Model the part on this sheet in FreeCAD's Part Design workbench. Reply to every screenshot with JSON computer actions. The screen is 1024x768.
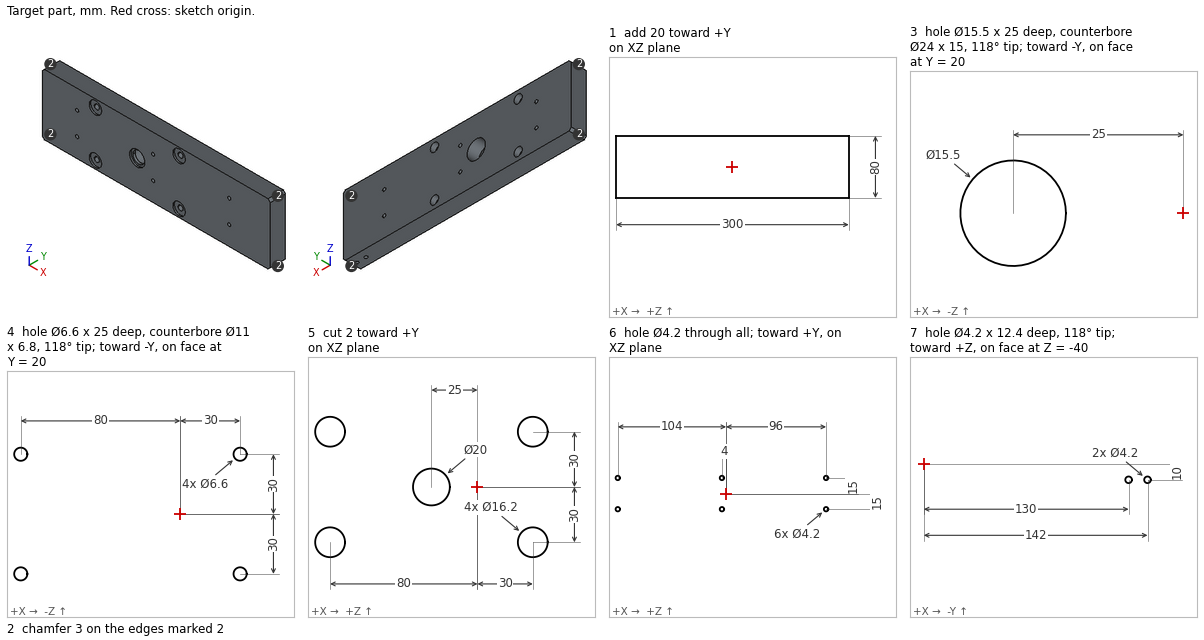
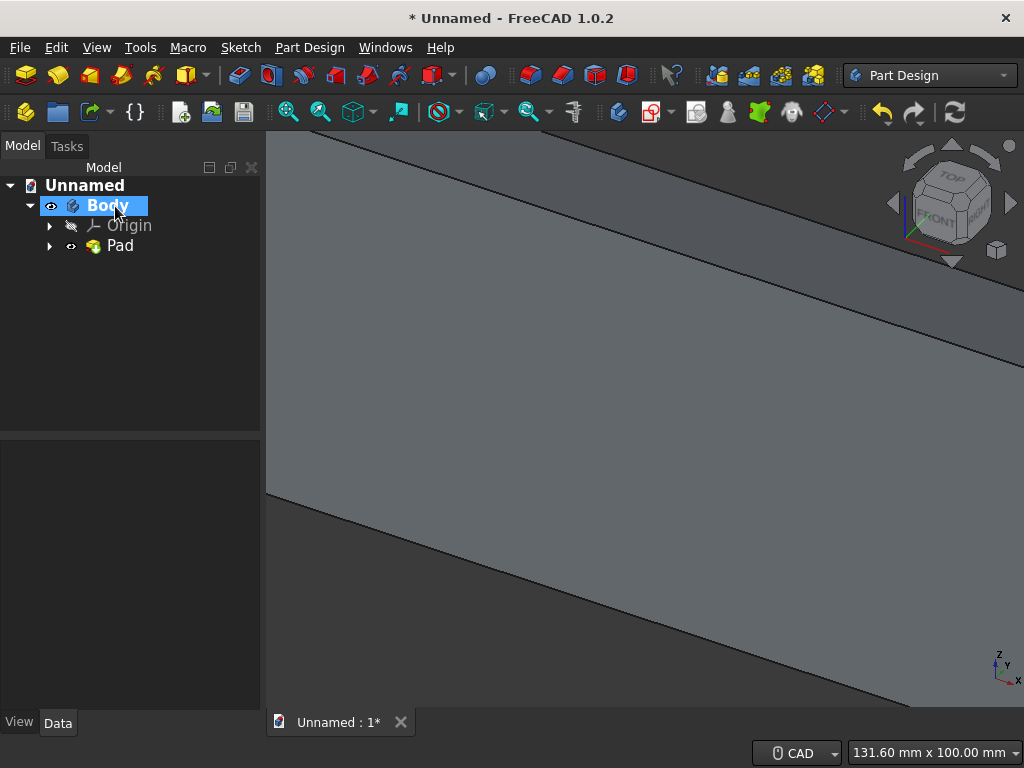
{"action": "left_click", "coordinate": [290, 112]}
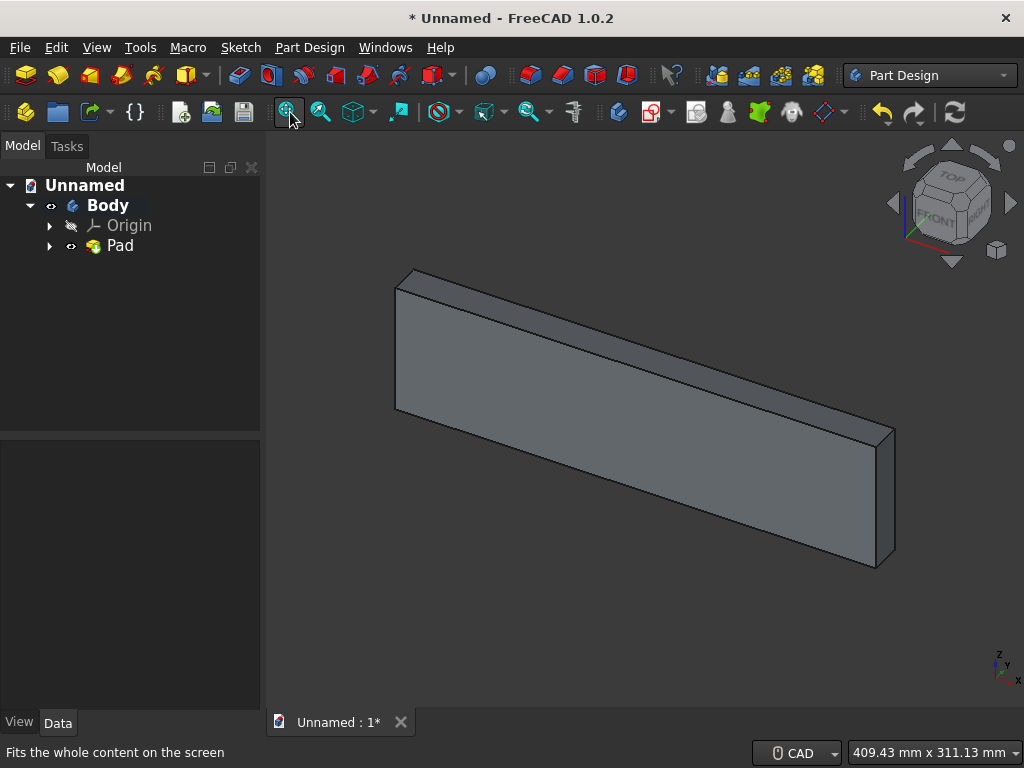
{"action": "left_click", "coordinate": [885, 437]}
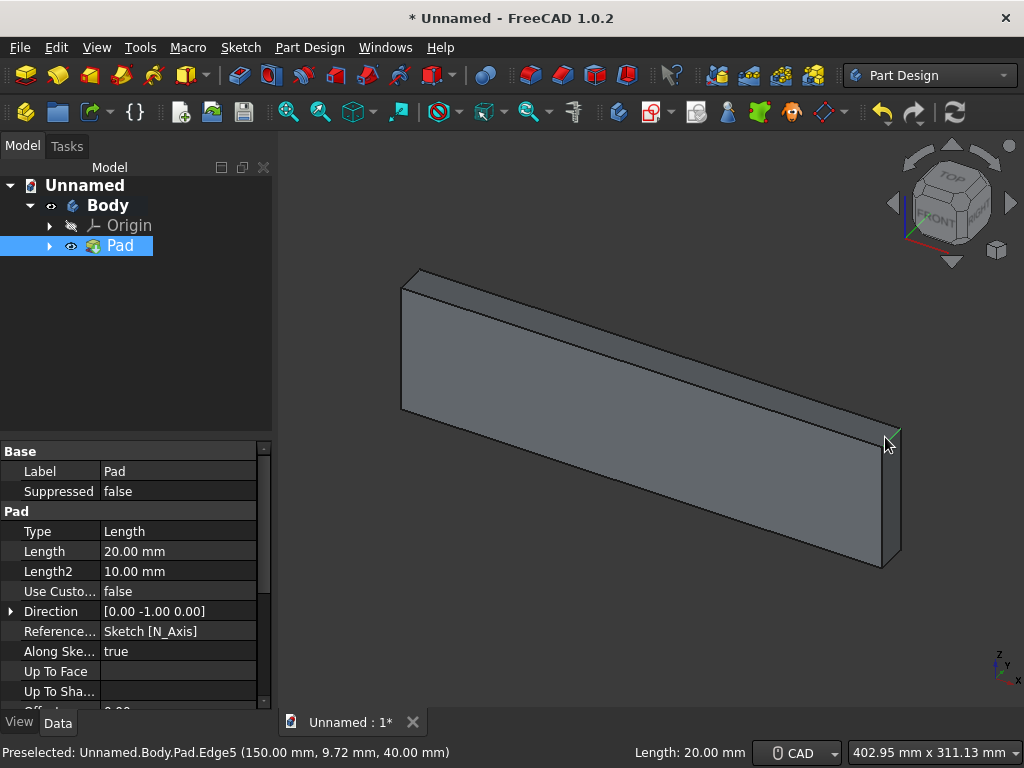
{"action": "key", "text": "0"}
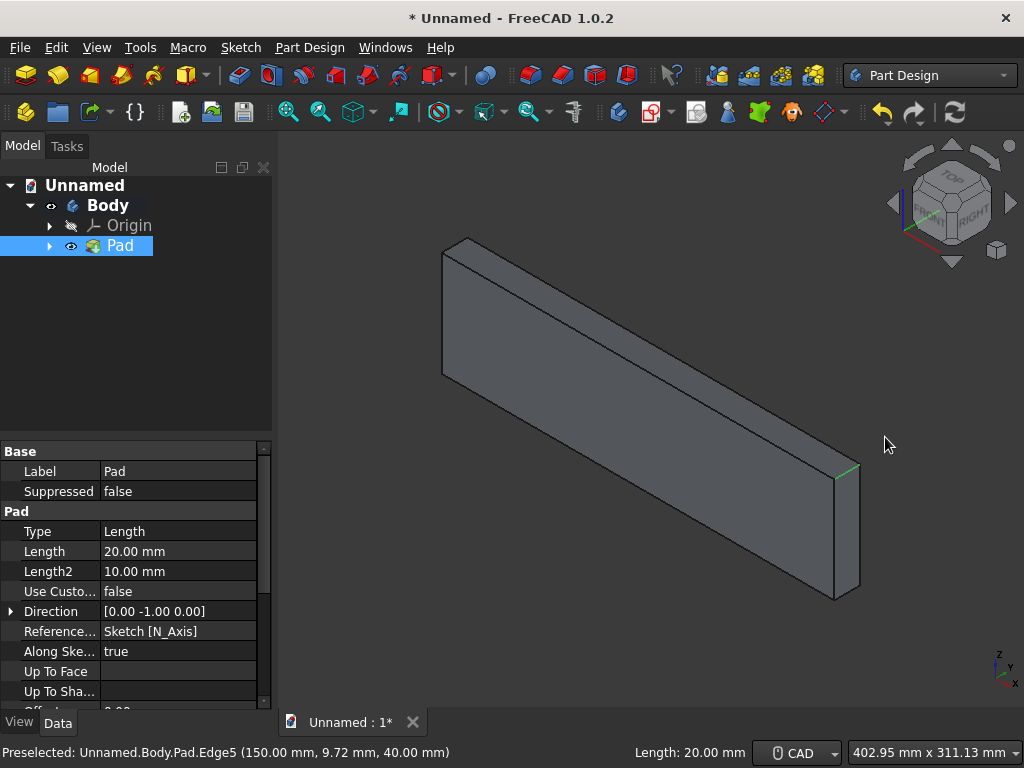
{"action": "key", "text": "2"}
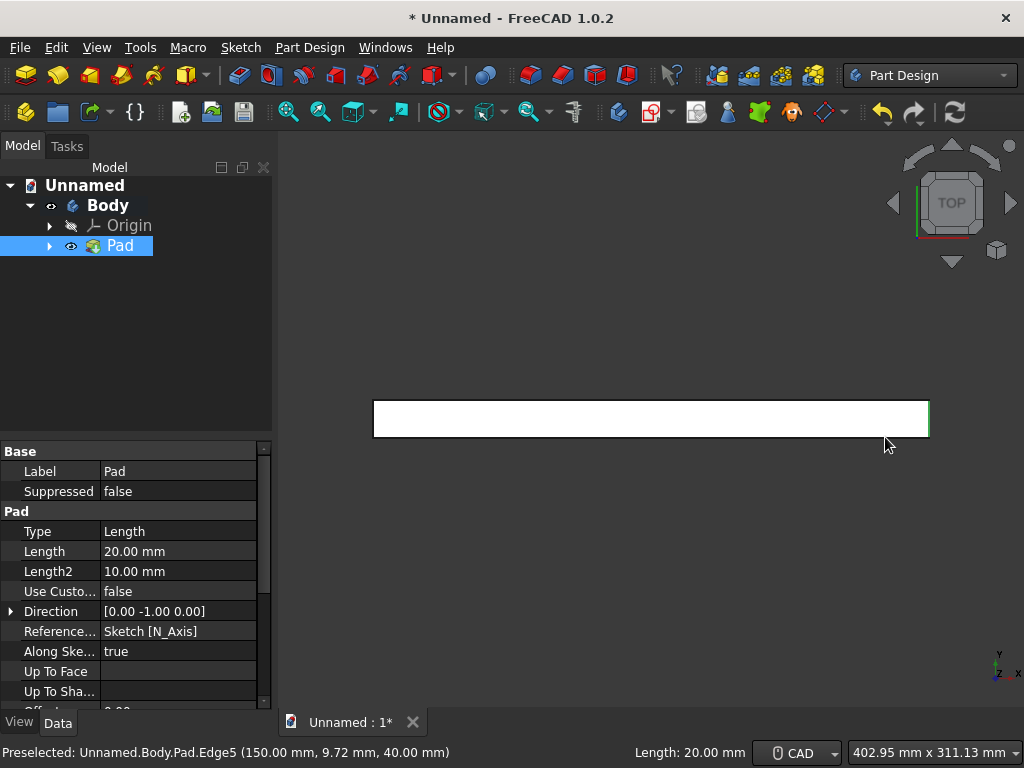
{"action": "left_click", "coordinate": [373, 418], "text": "ctrl"}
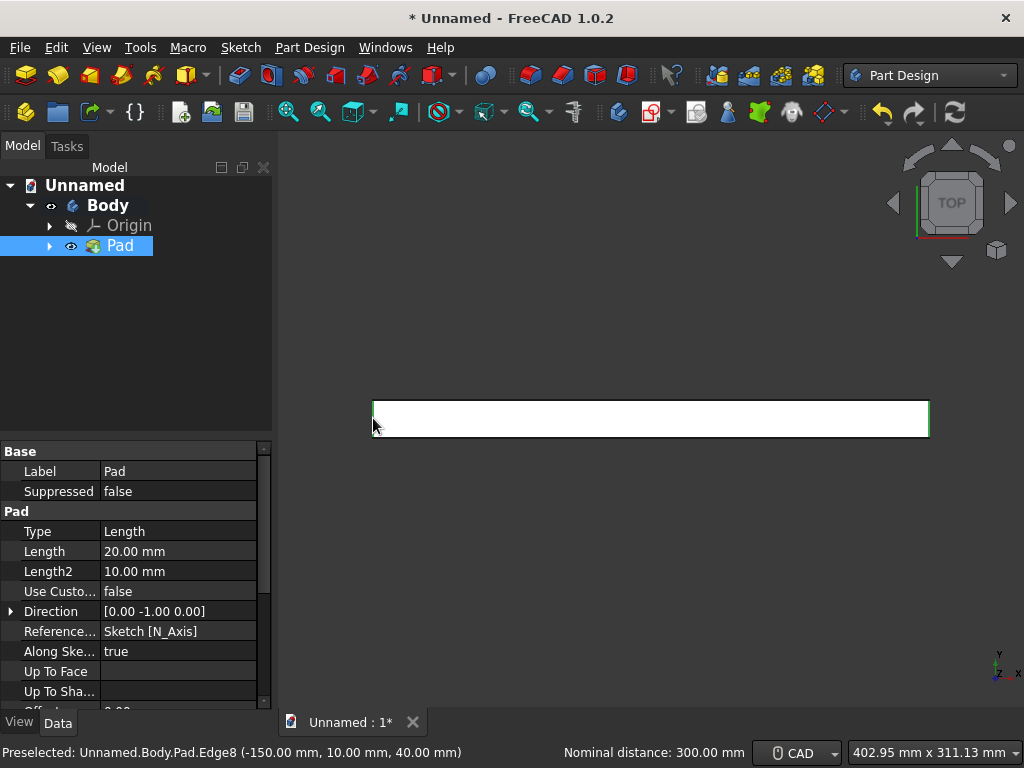
{"action": "key", "text": "1"}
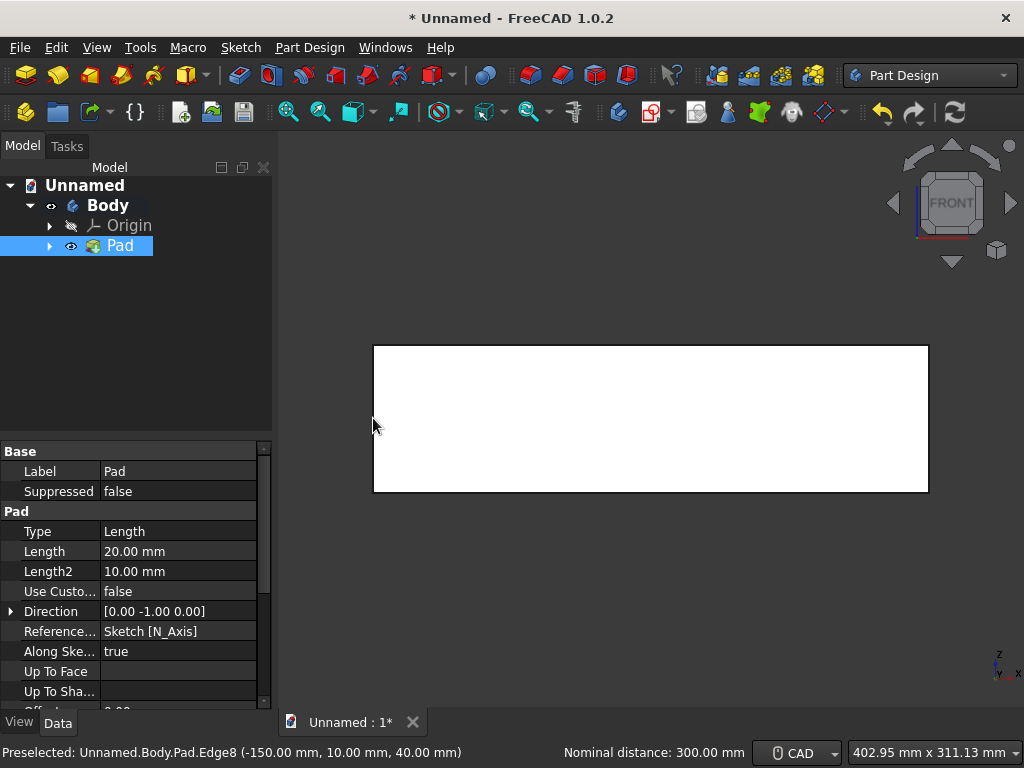
{"action": "key", "text": "3"}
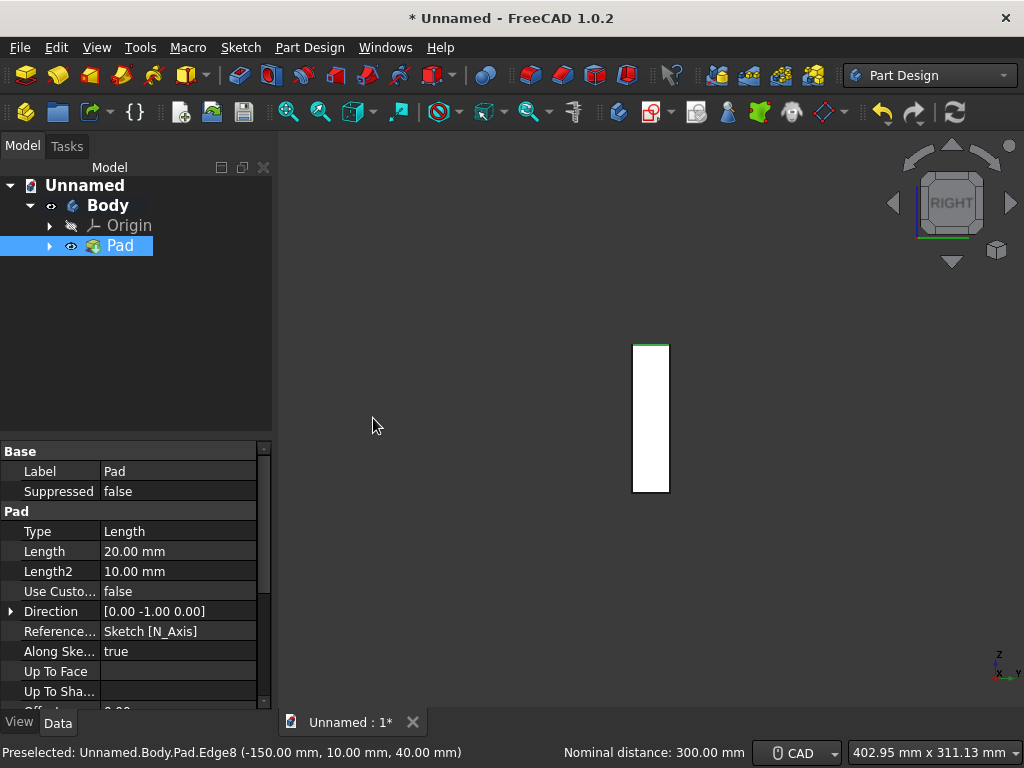
{"action": "left_click", "coordinate": [290, 112]}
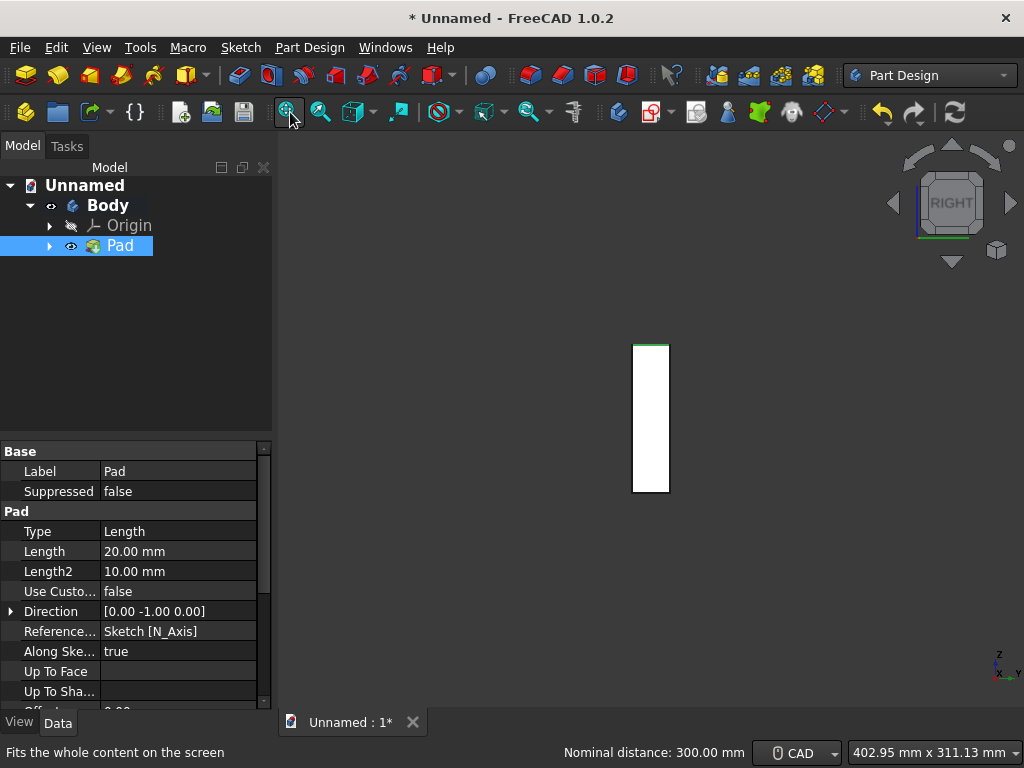
{"action": "left_click", "coordinate": [651, 492], "text": "ctrl"}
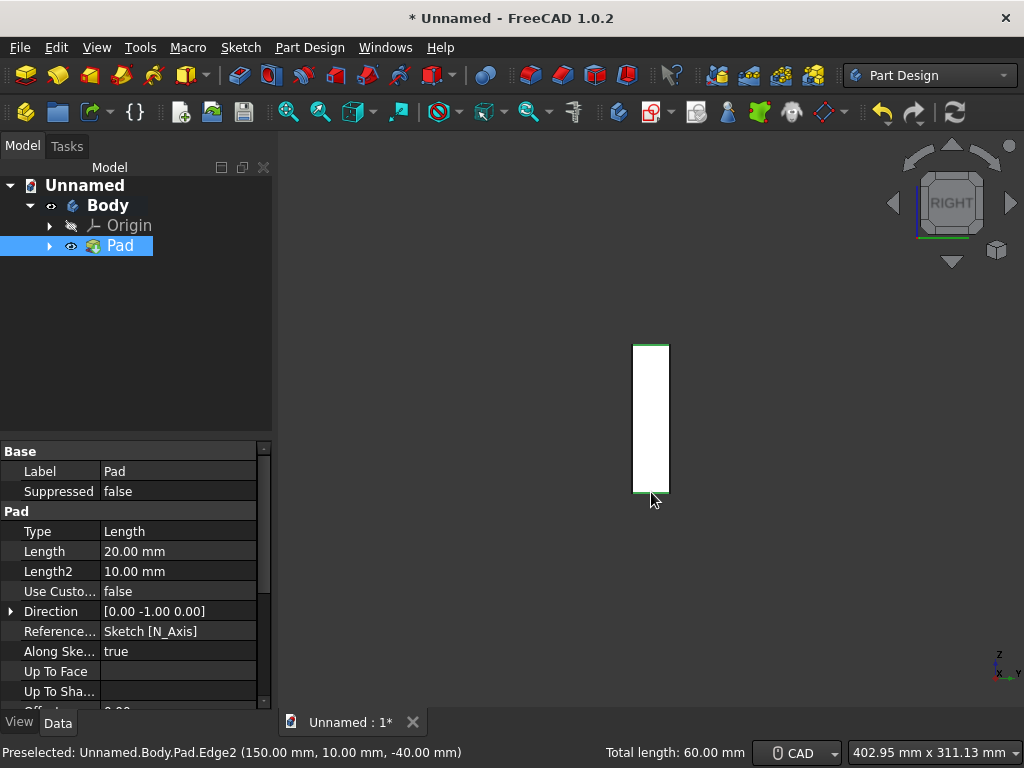
{"action": "key", "text": "5"}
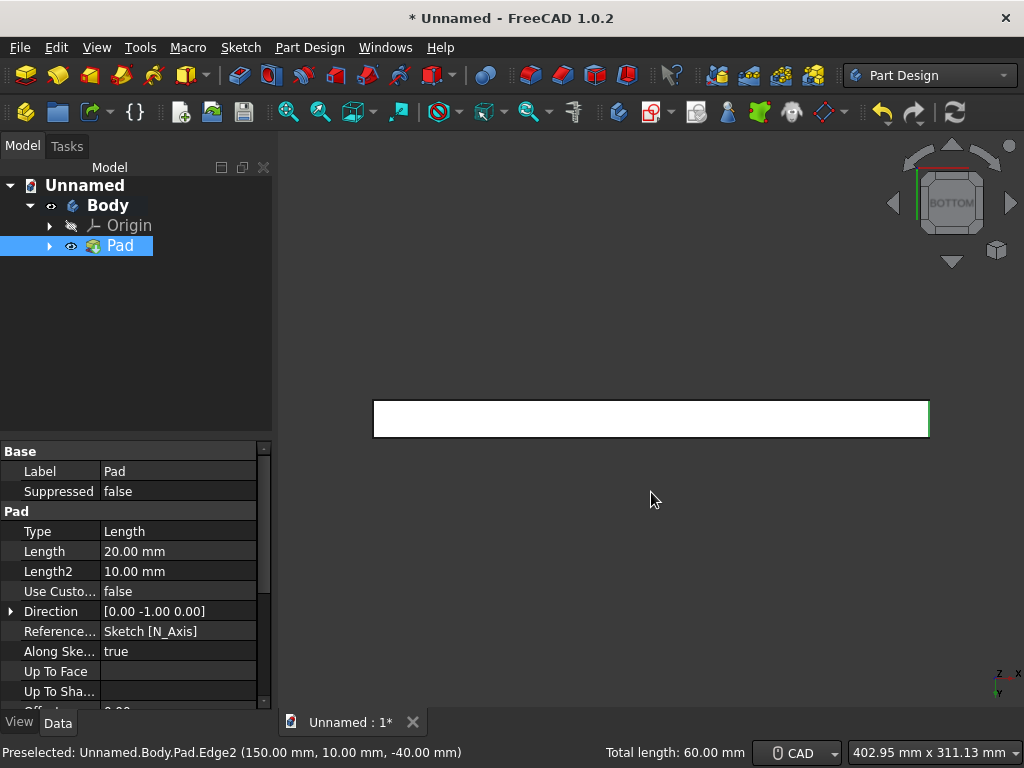
{"action": "left_click", "coordinate": [373, 418], "text": "ctrl"}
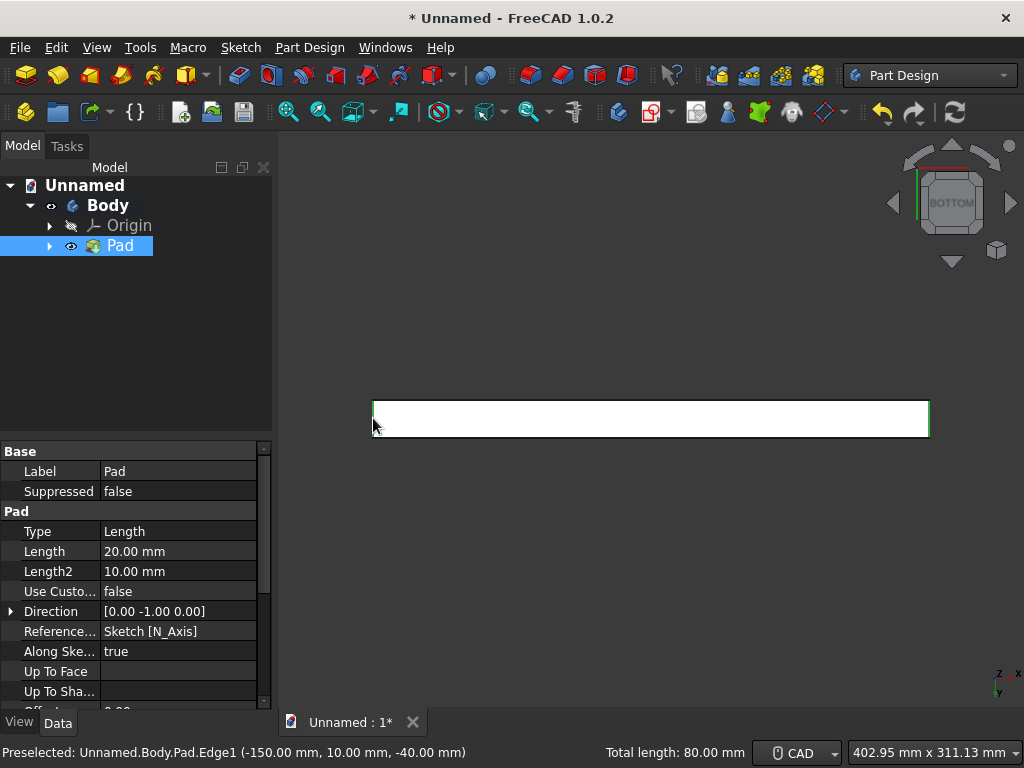
{"action": "left_click", "coordinate": [564, 76]}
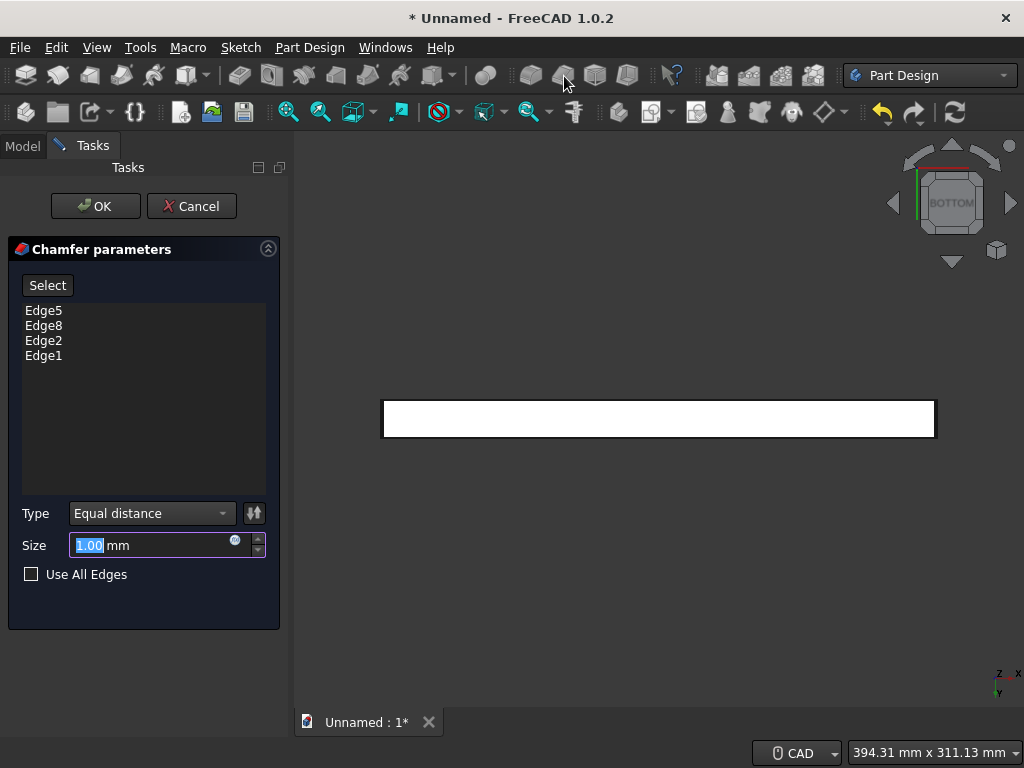
{"action": "type", "text": "3"}
{"action": "key", "text": "Tab"}